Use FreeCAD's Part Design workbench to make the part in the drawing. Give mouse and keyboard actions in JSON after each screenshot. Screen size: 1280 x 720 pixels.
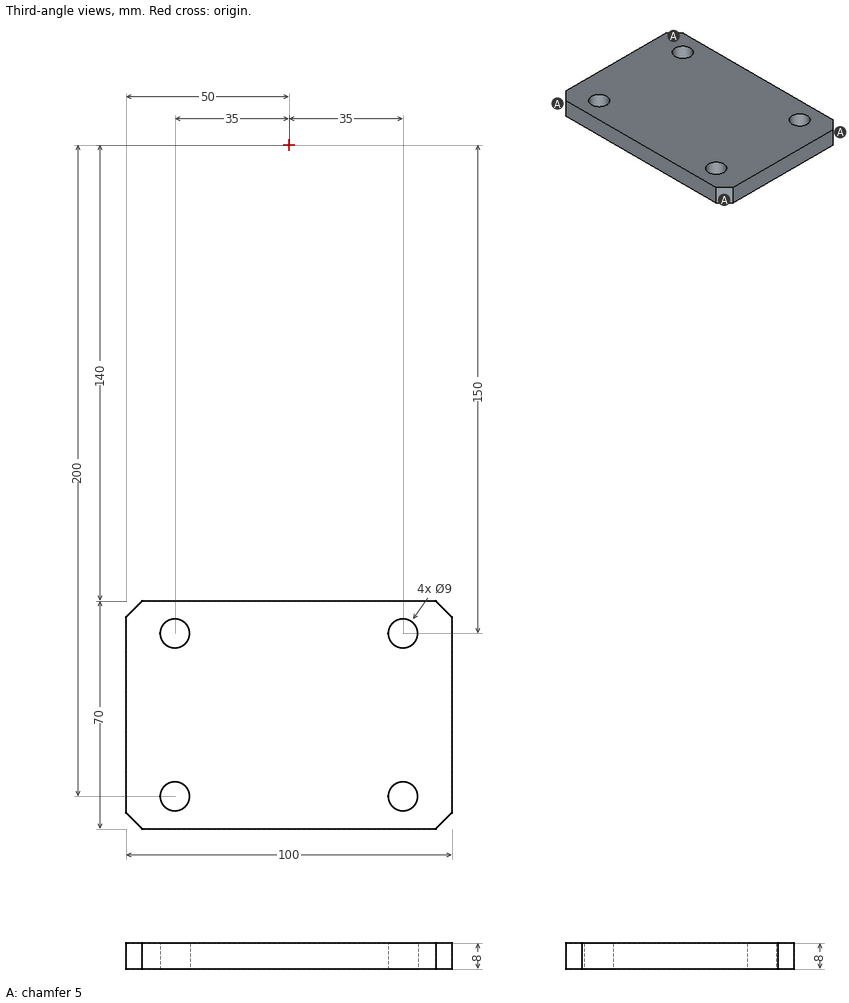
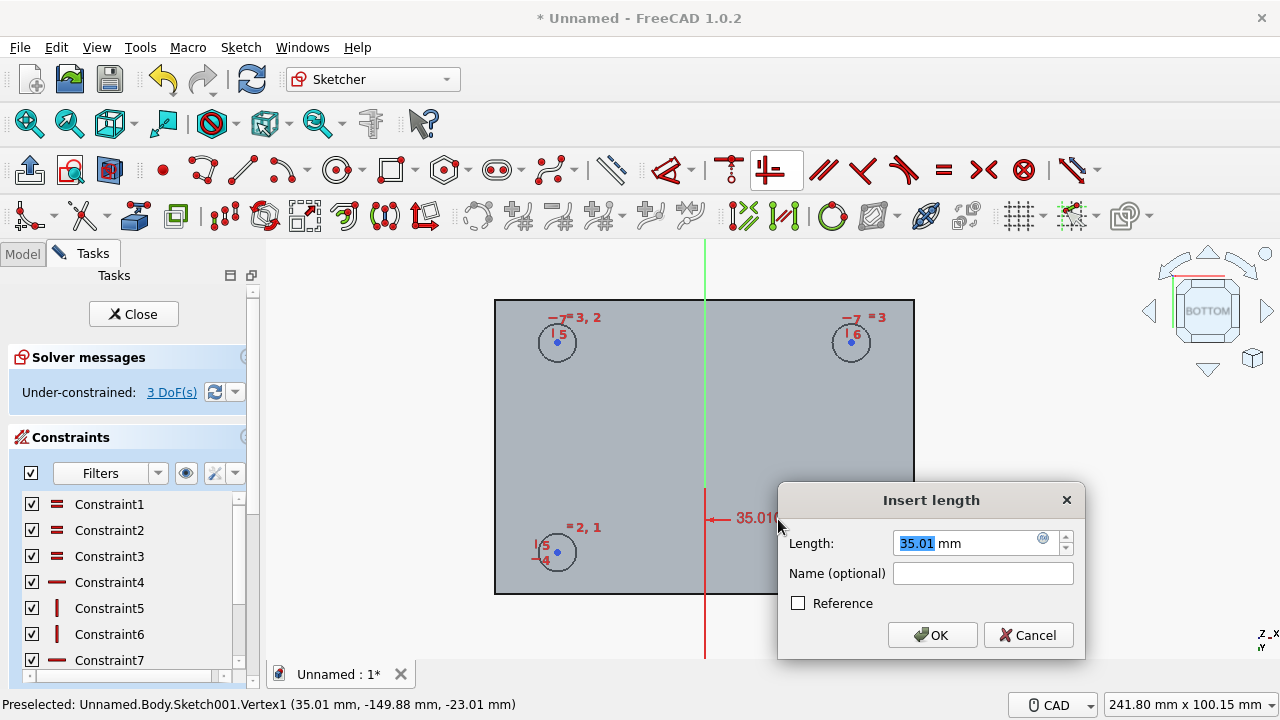
{"action": "type", "text": "35"}
{"action": "key", "text": "Return"}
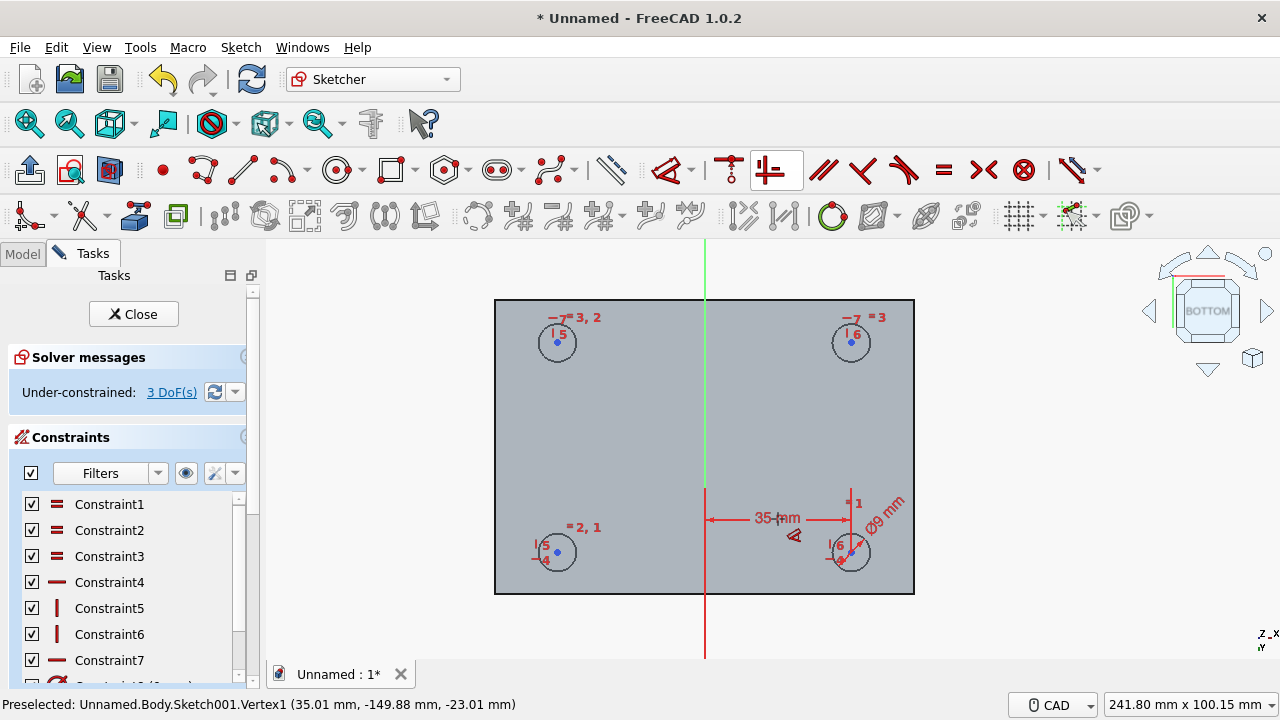
{"action": "left_click", "coordinate": [557, 553]}
{"action": "left_click", "coordinate": [631, 519]}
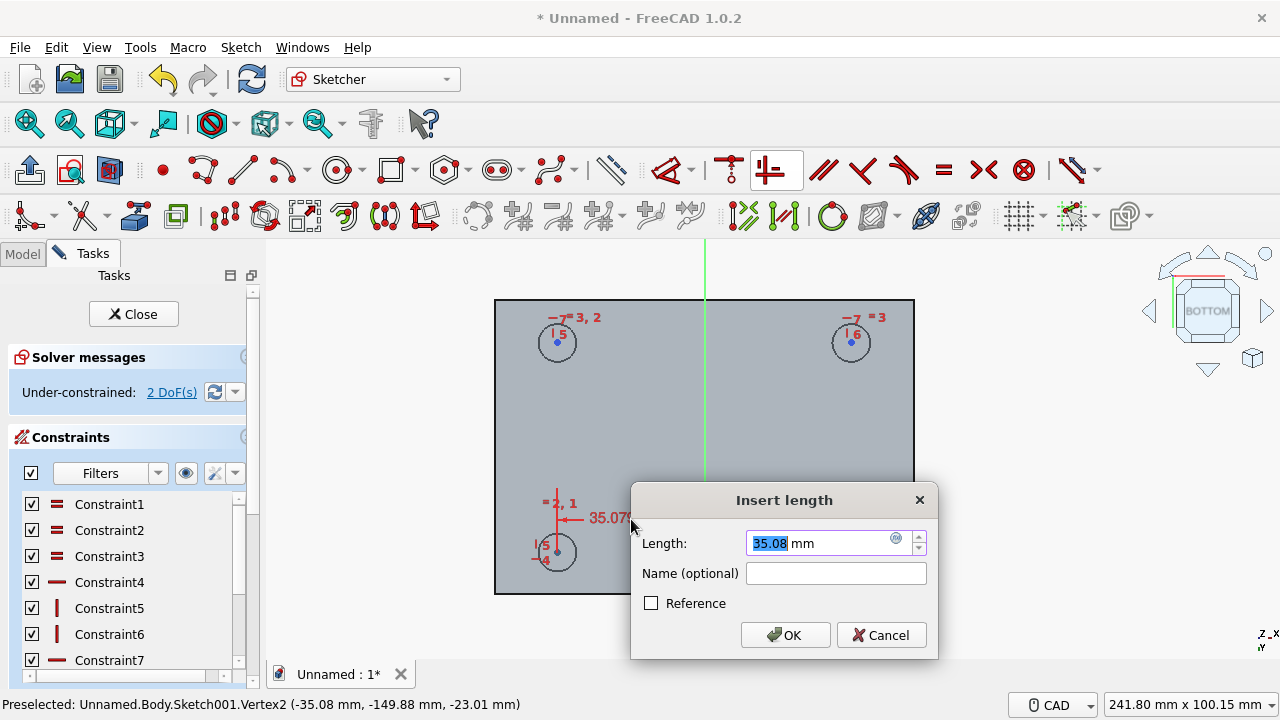
{"action": "type", "text": "35"}
{"action": "key", "text": "Return"}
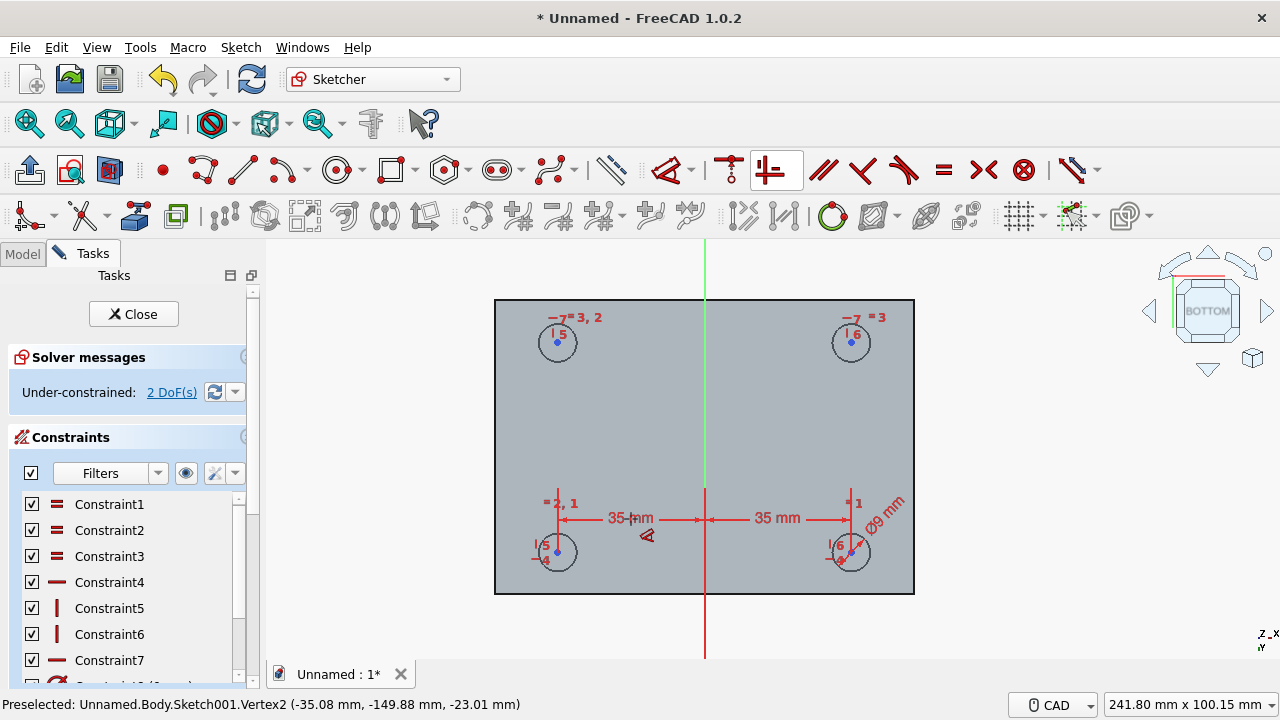
{"action": "left_click", "coordinate": [851, 553]}
{"action": "left_click", "coordinate": [885, 592]}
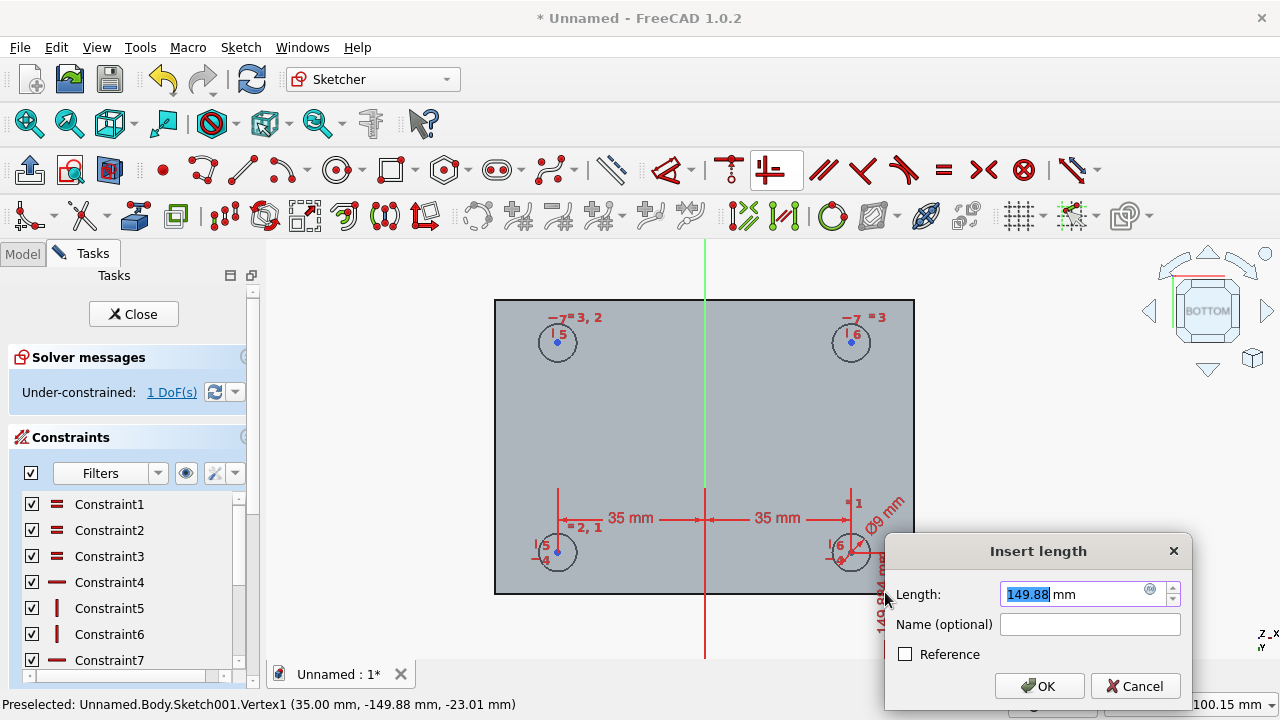
{"action": "type", "text": "150"}
{"action": "key", "text": "Return"}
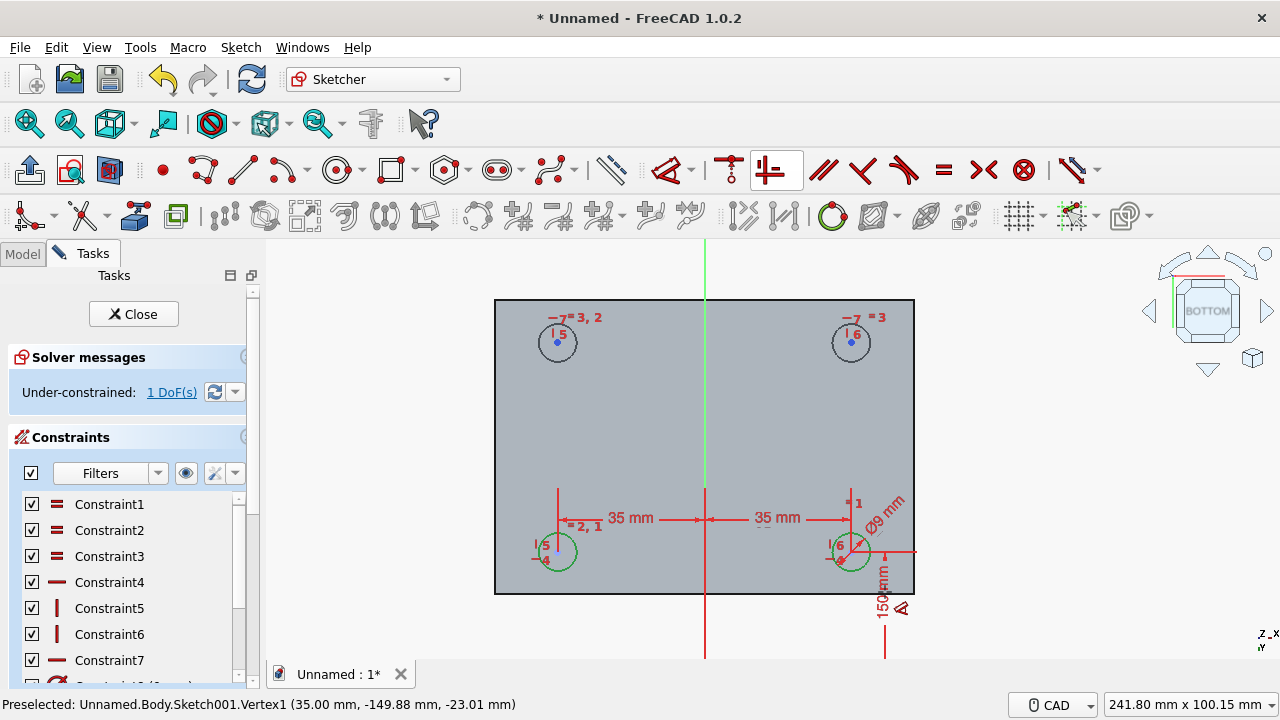
{"action": "left_click", "coordinate": [558, 343]}
{"action": "left_click", "coordinate": [524, 487]}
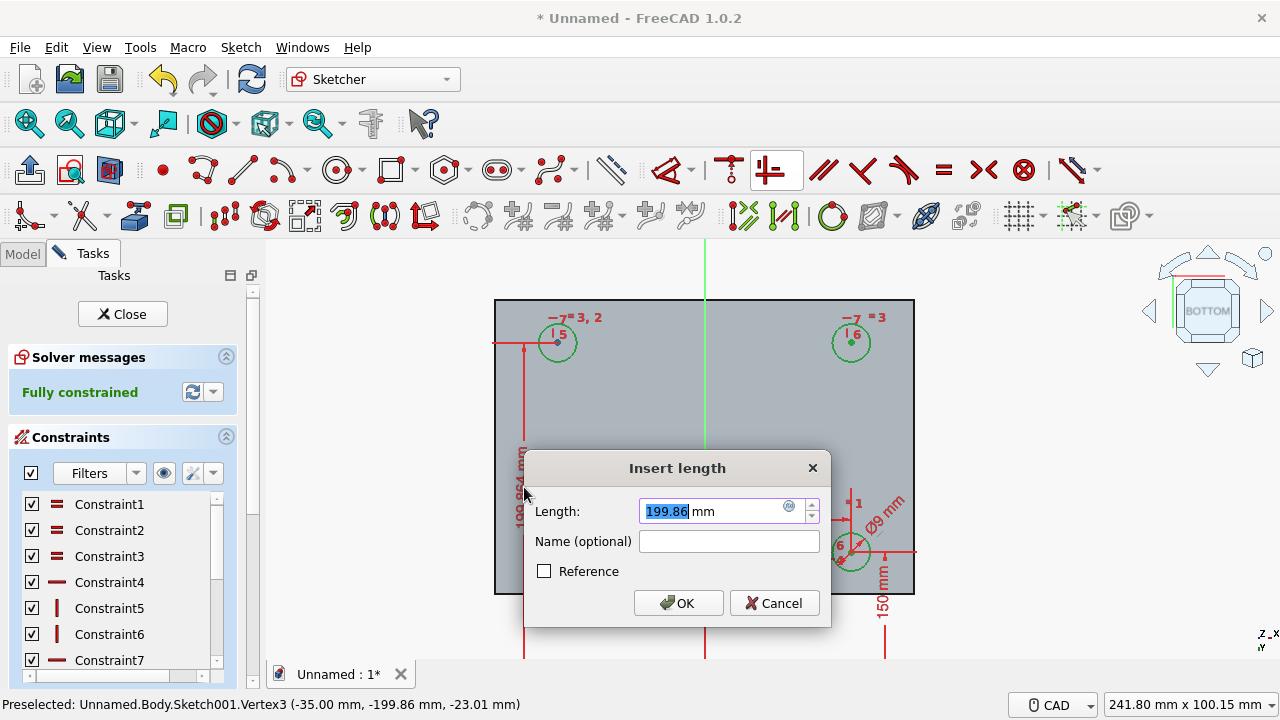
{"action": "type", "text": "200"}
{"action": "key", "text": "Return"}
{"action": "key", "text": "Escape"}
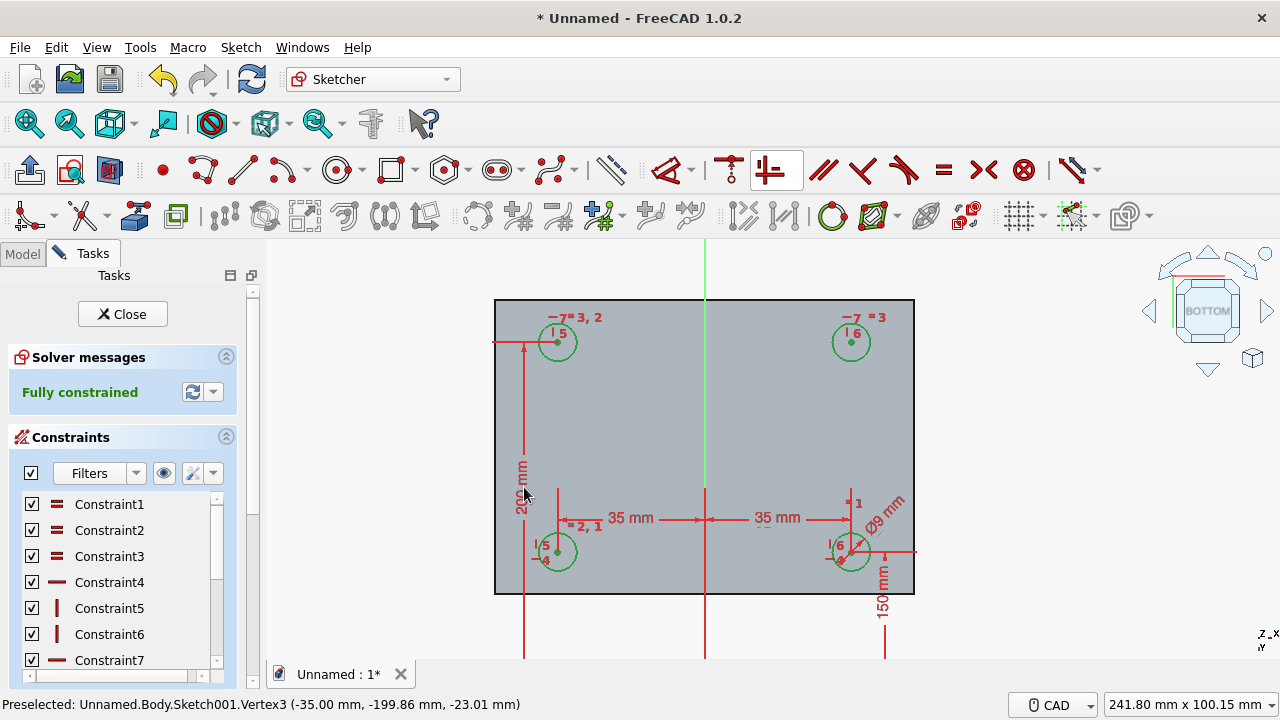
{"action": "left_click", "coordinate": [123, 314]}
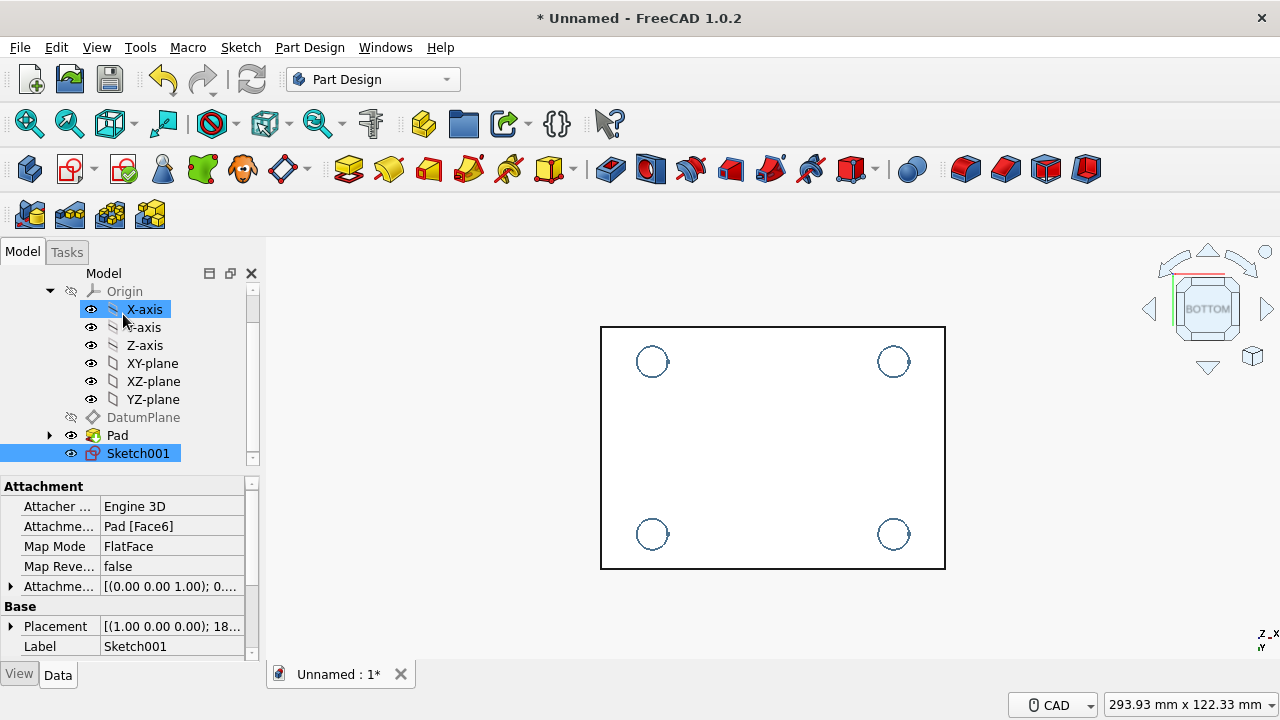
{"action": "left_click", "coordinate": [612, 170]}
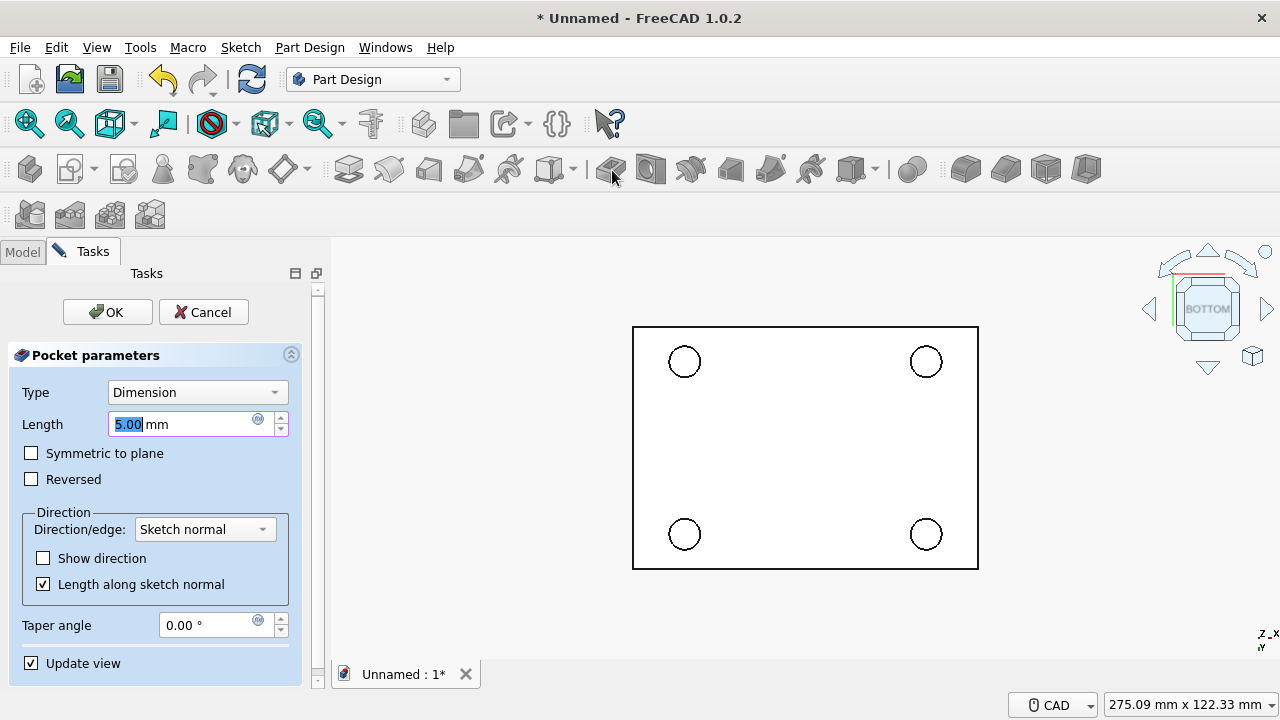
{"action": "type", "text": "8"}
{"action": "key", "text": "Tab"}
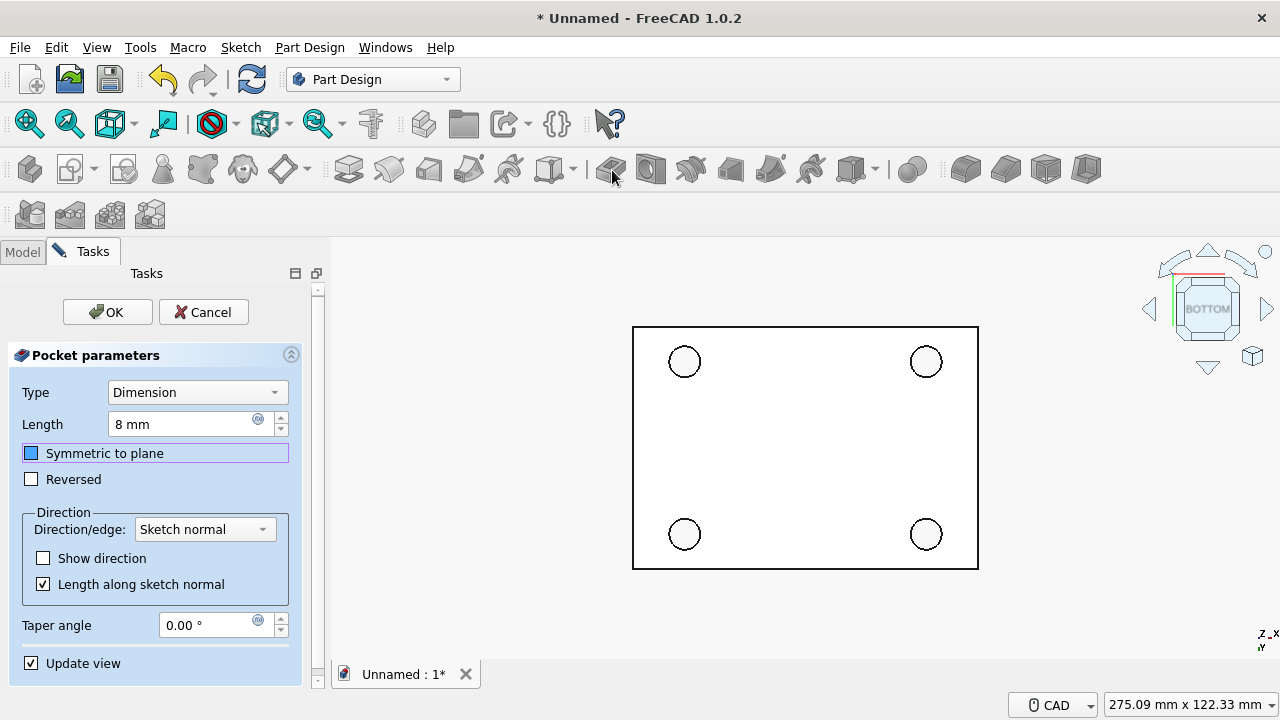
{"action": "left_click", "coordinate": [108, 312]}